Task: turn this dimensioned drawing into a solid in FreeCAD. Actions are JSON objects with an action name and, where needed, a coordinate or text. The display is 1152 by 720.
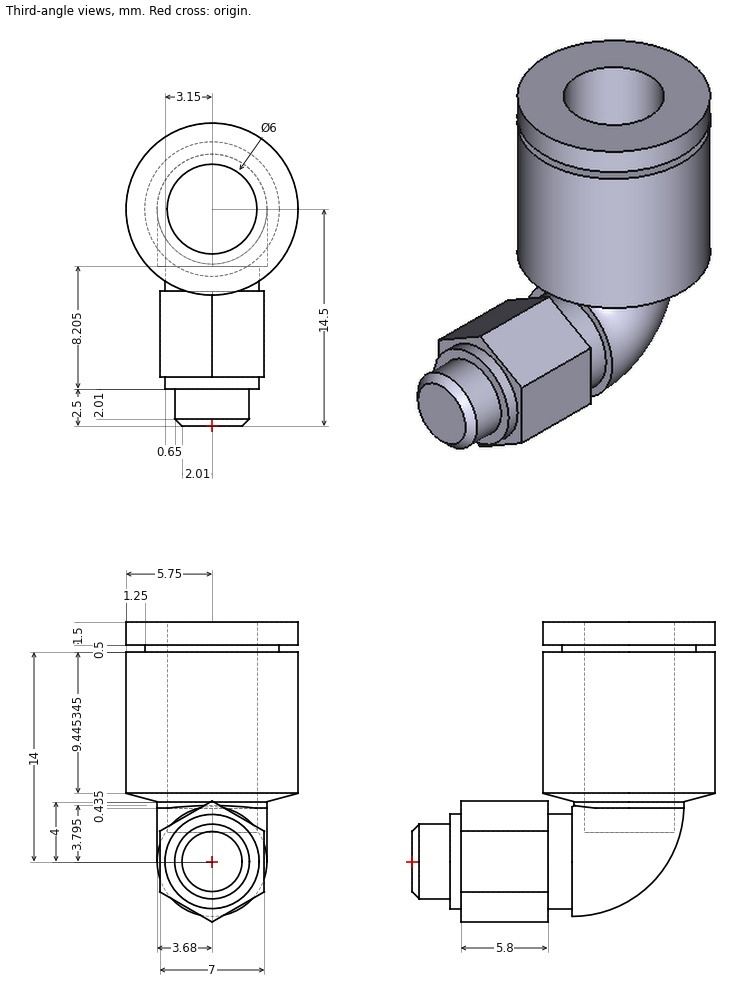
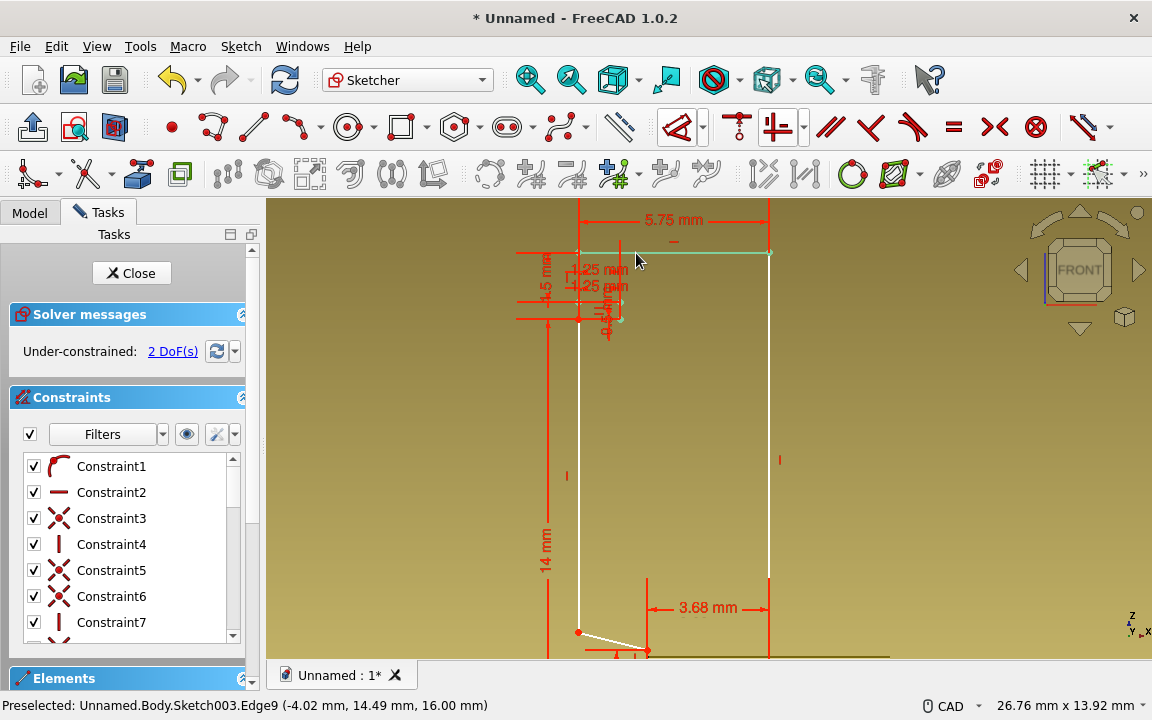
{"action": "scroll", "coordinate": [600, 320], "scroll_direction": "down", "scroll_amount": 3}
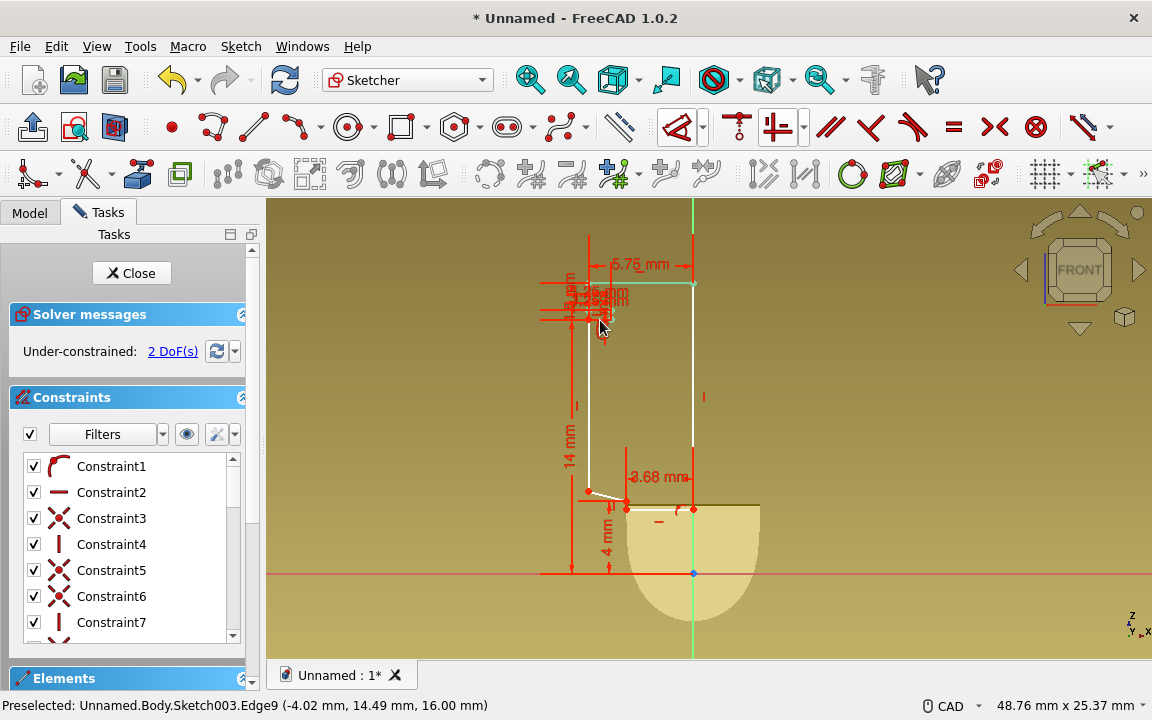
{"action": "scroll", "coordinate": [626, 506], "scroll_direction": "up", "scroll_amount": 9}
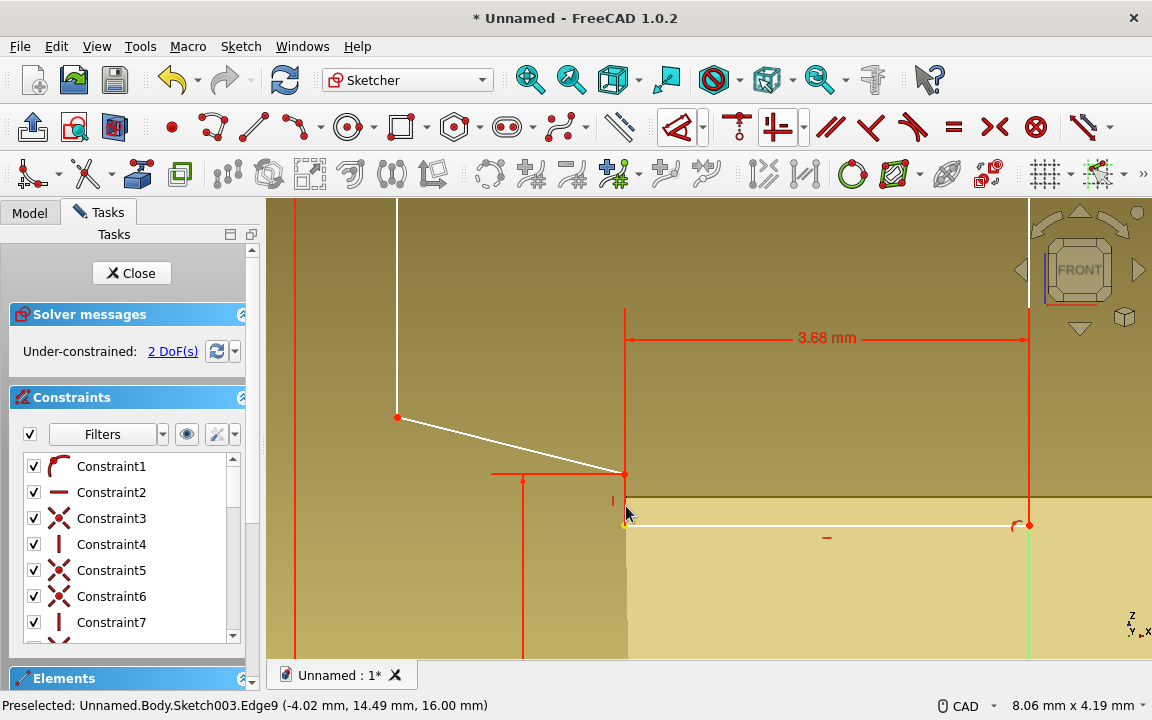
{"action": "left_click", "coordinate": [625, 500]}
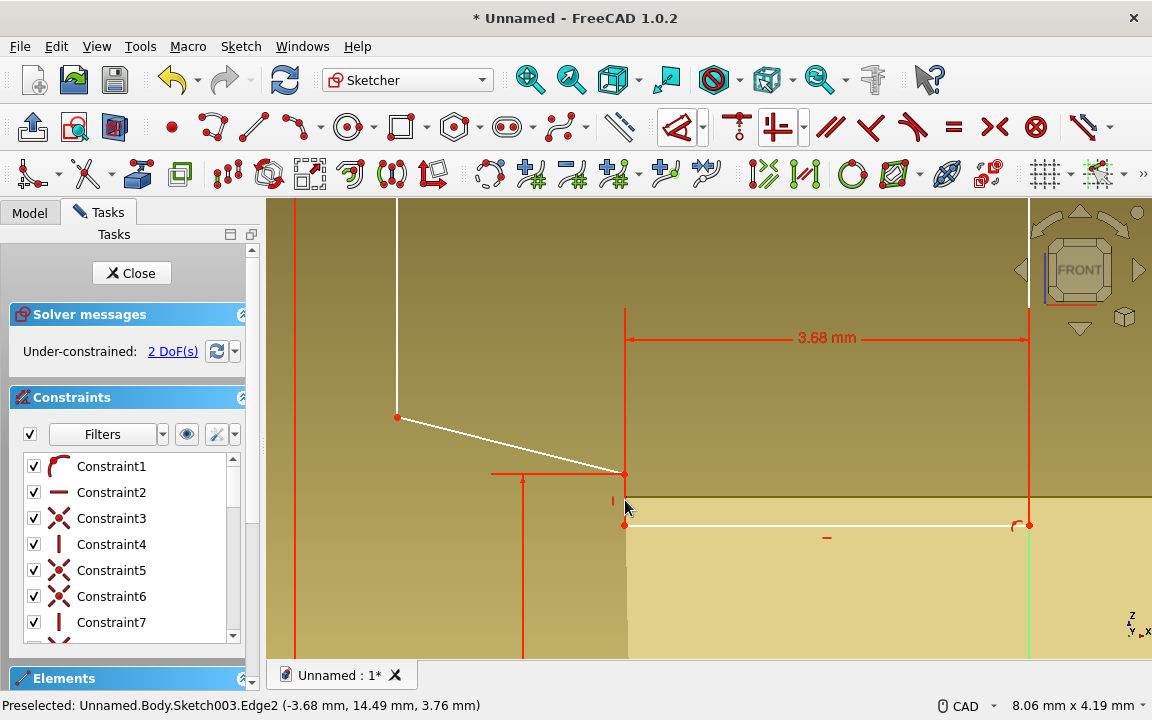
{"action": "key", "text": "i"}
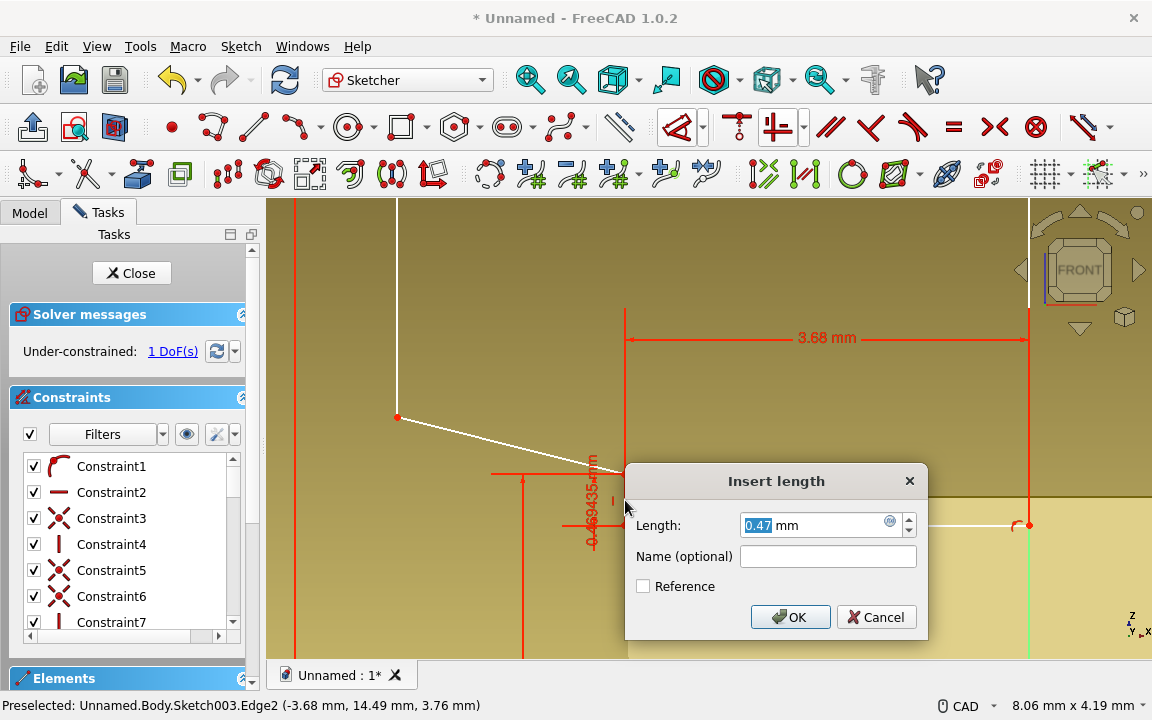
{"action": "type", "text": "0.435"}
{"action": "key", "text": "Return"}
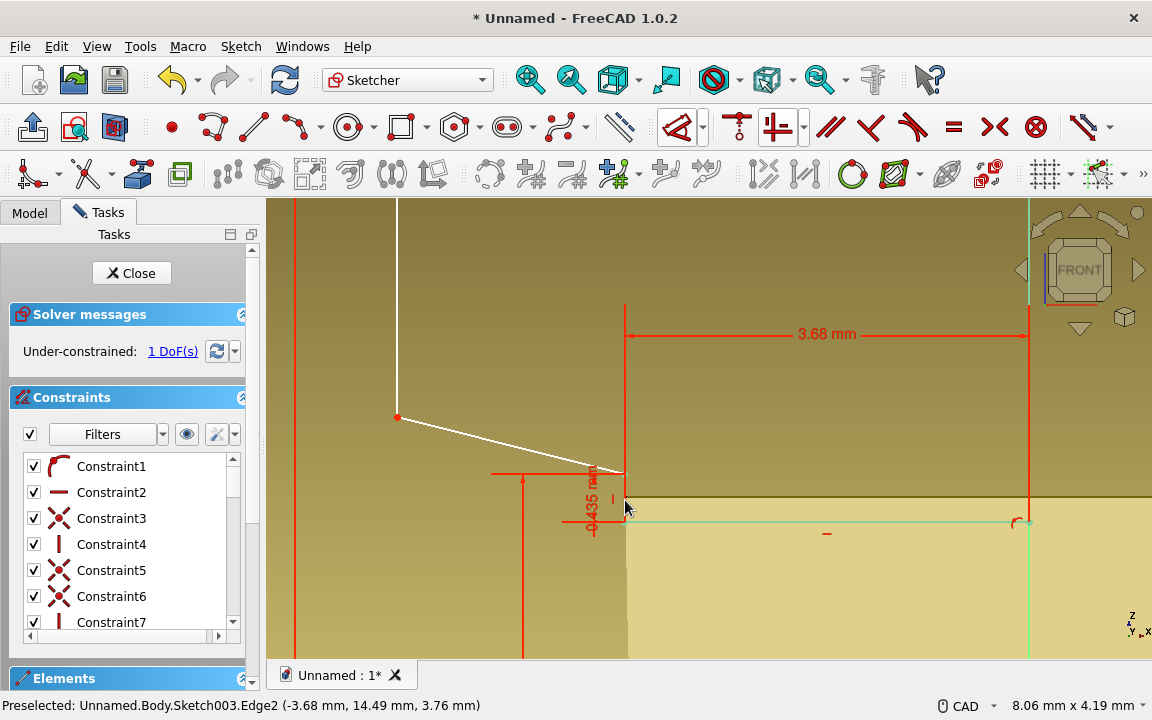
{"action": "scroll", "coordinate": [626, 507], "scroll_direction": "down", "scroll_amount": 9}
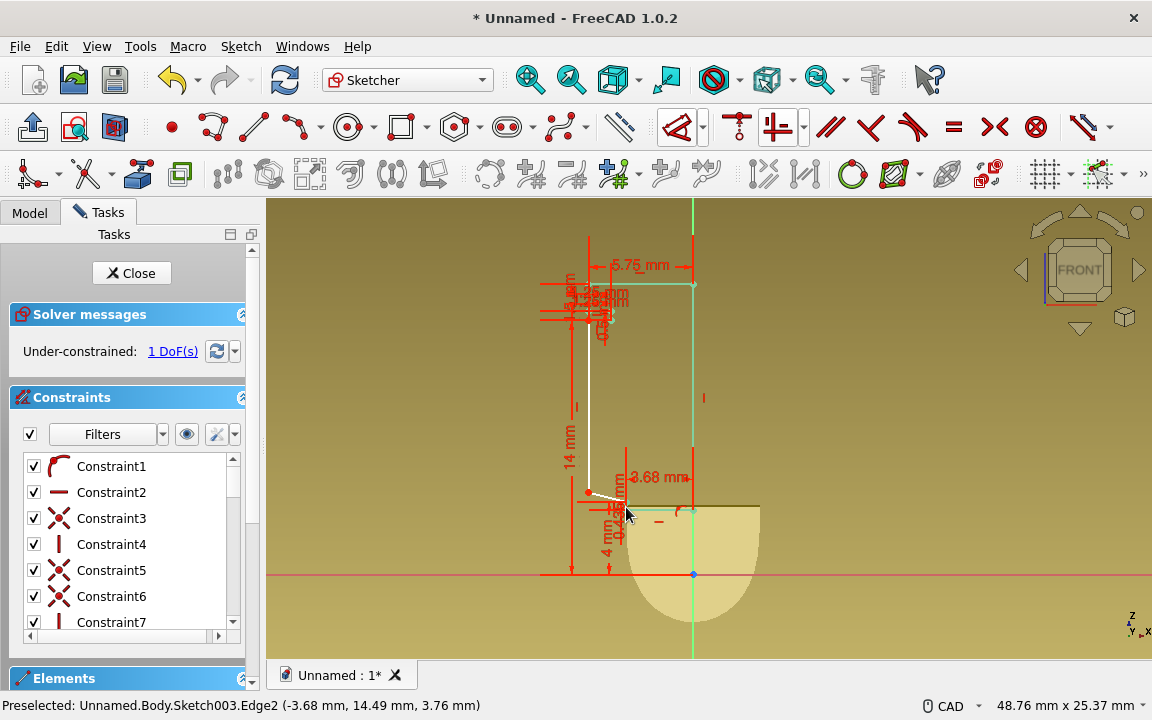
{"action": "left_click", "coordinate": [589, 441]}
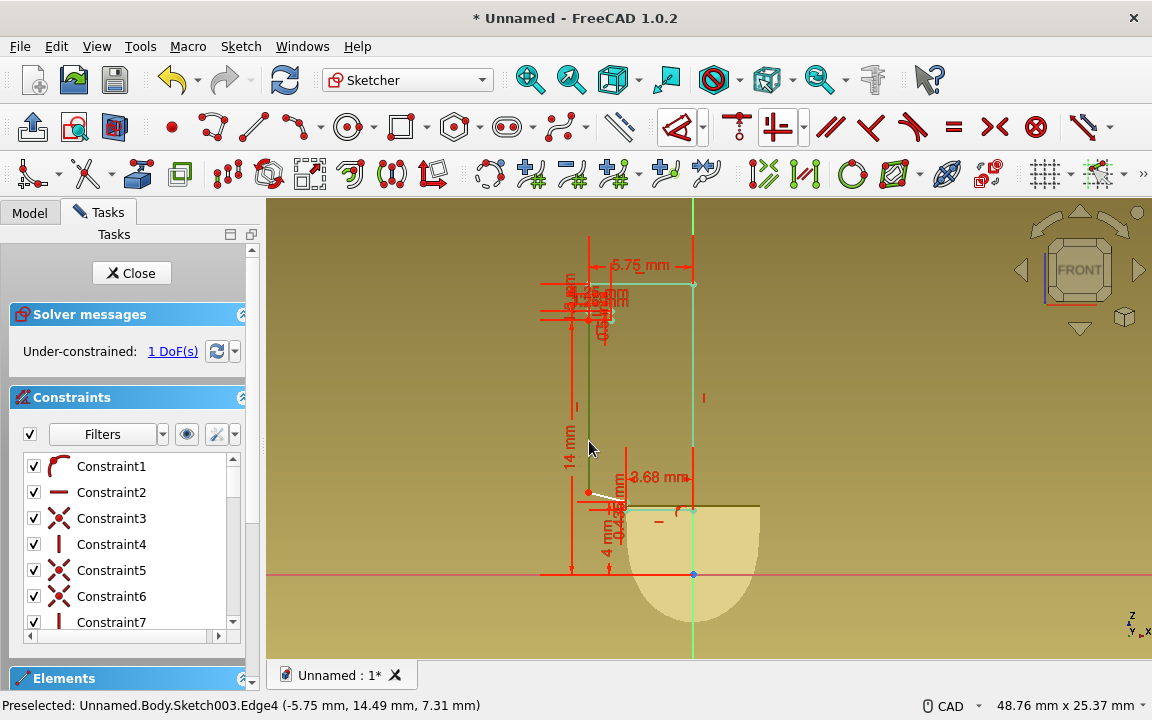
{"action": "key", "text": "i"}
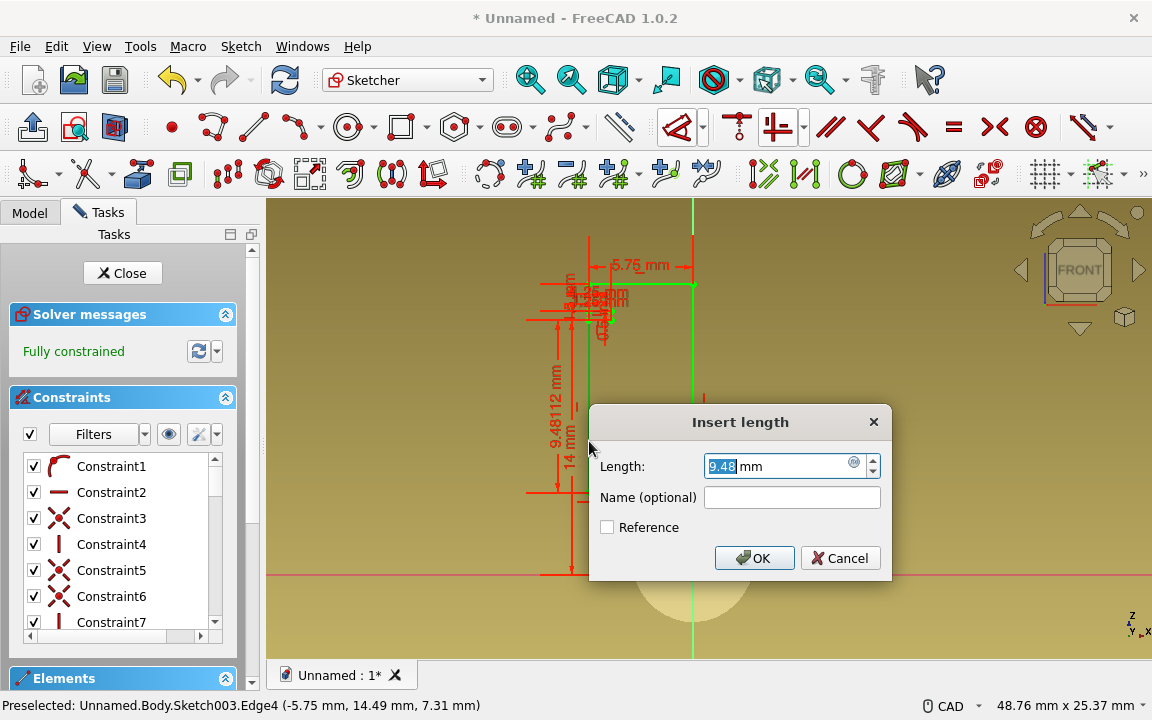
{"action": "type", "text": "9.445345"}
{"action": "key", "text": "Return"}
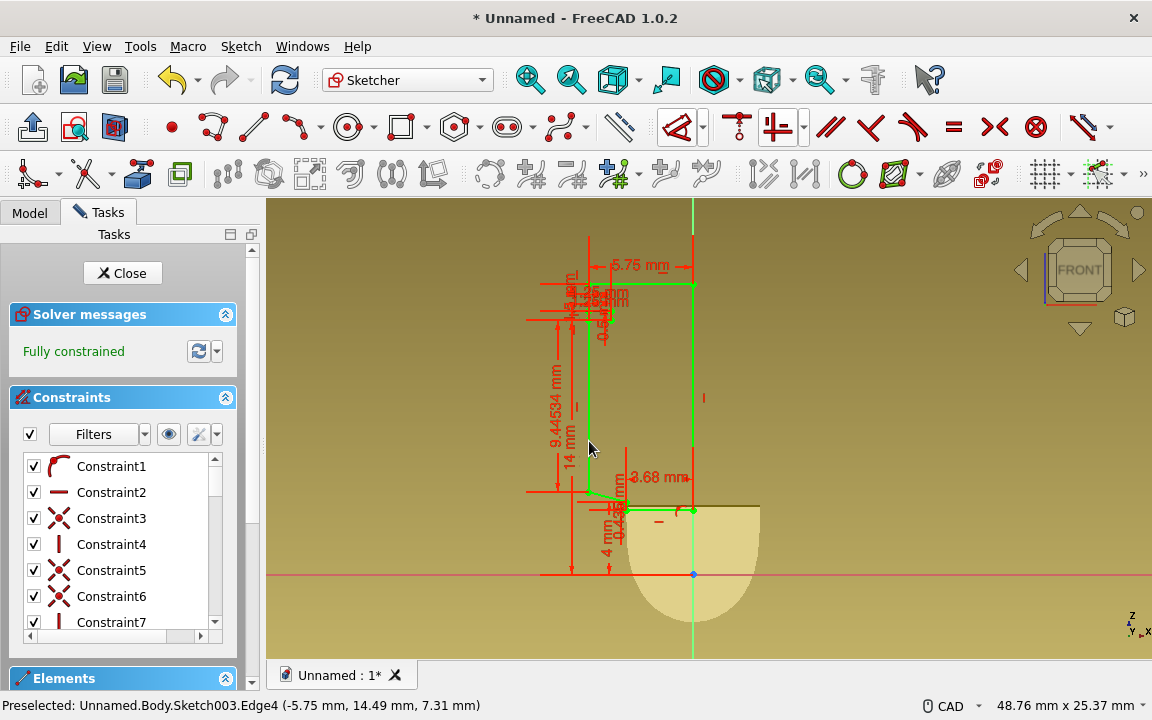
{"action": "left_click", "coordinate": [123, 273]}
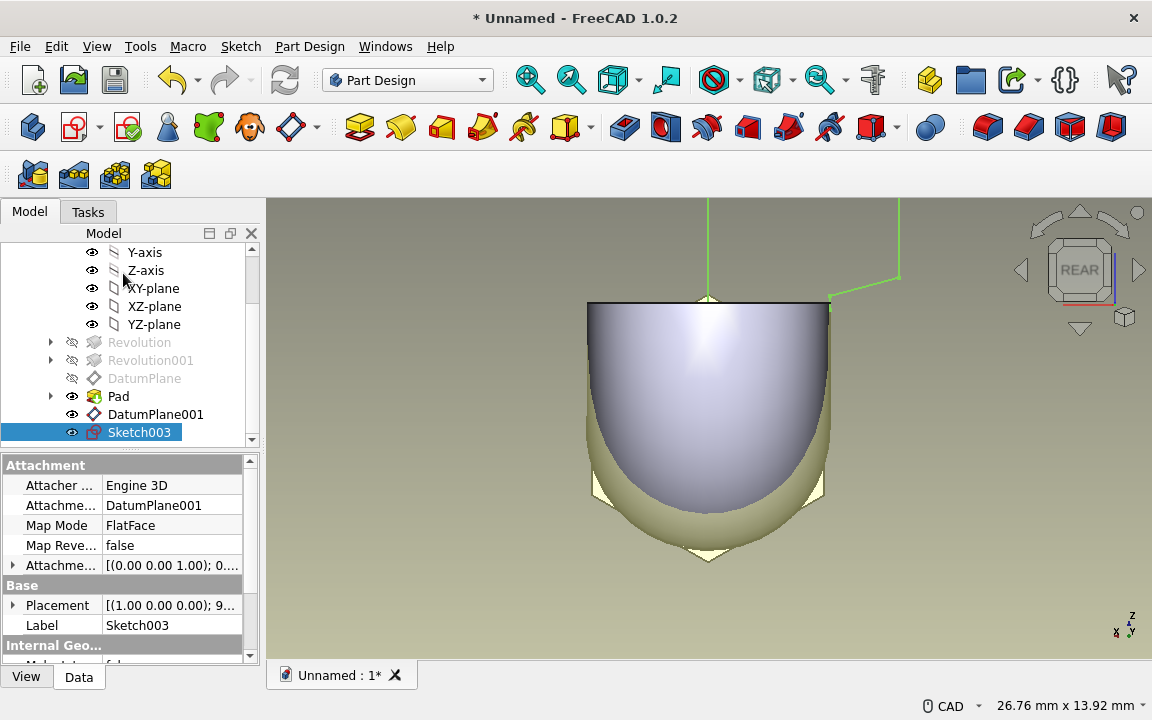
{"action": "left_click", "coordinate": [401, 128]}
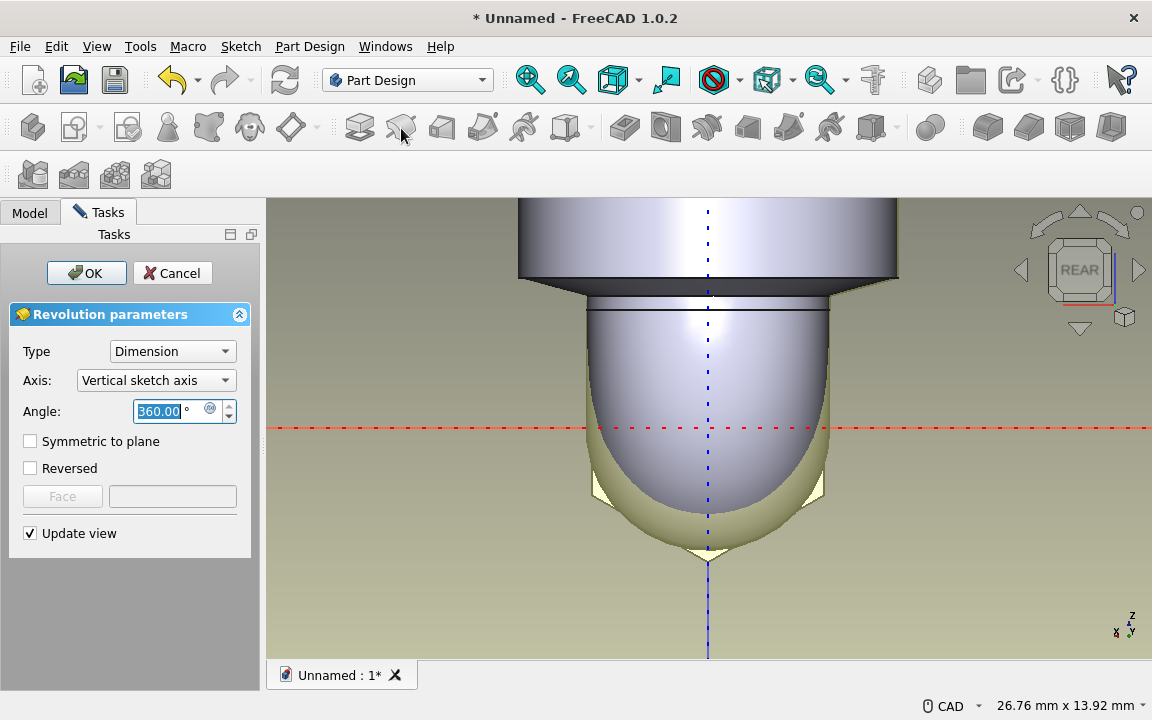
{"action": "left_click", "coordinate": [87, 273]}